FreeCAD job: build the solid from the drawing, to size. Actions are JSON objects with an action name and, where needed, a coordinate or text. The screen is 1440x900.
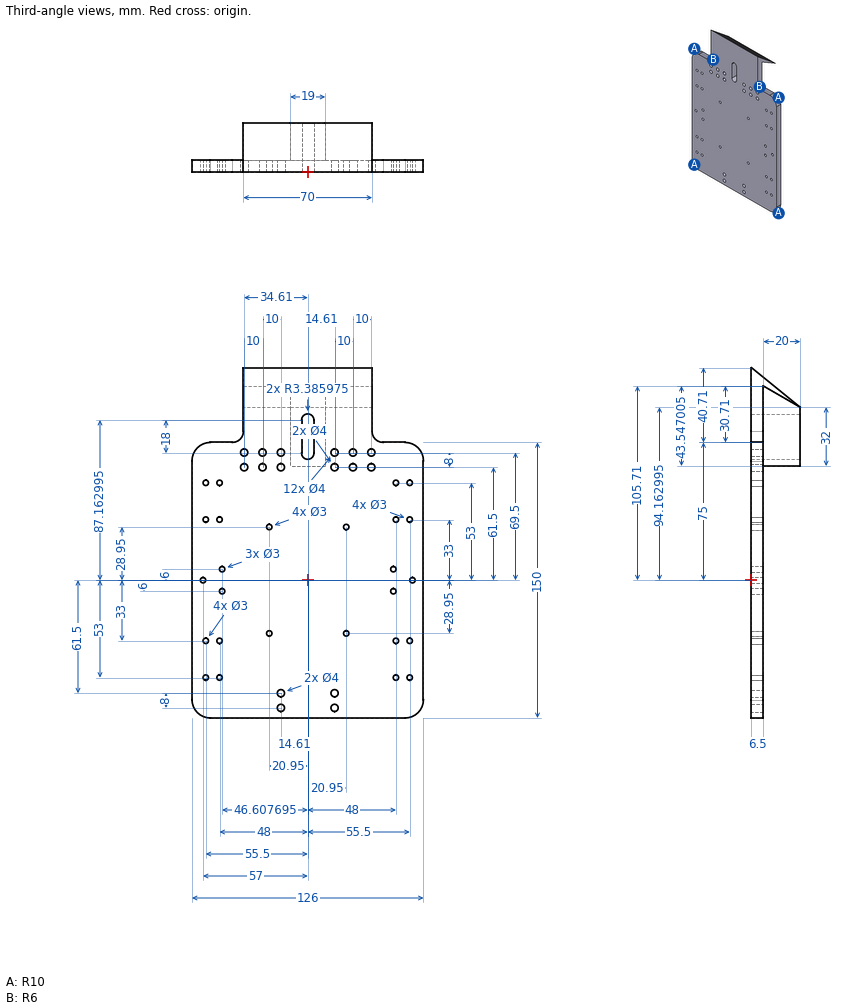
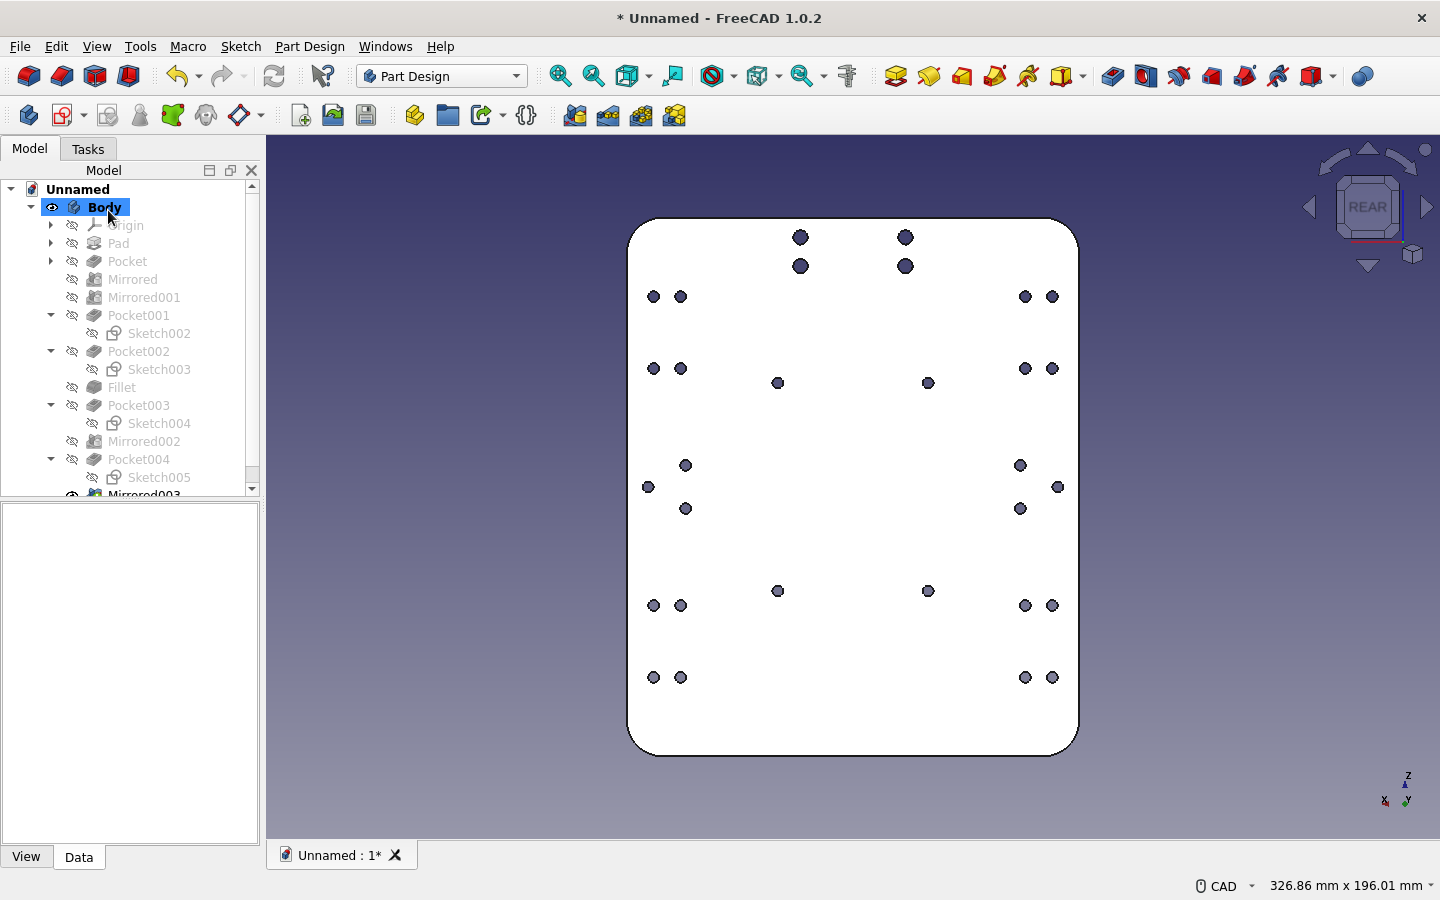
{"action": "left_click", "coordinate": [117, 459]}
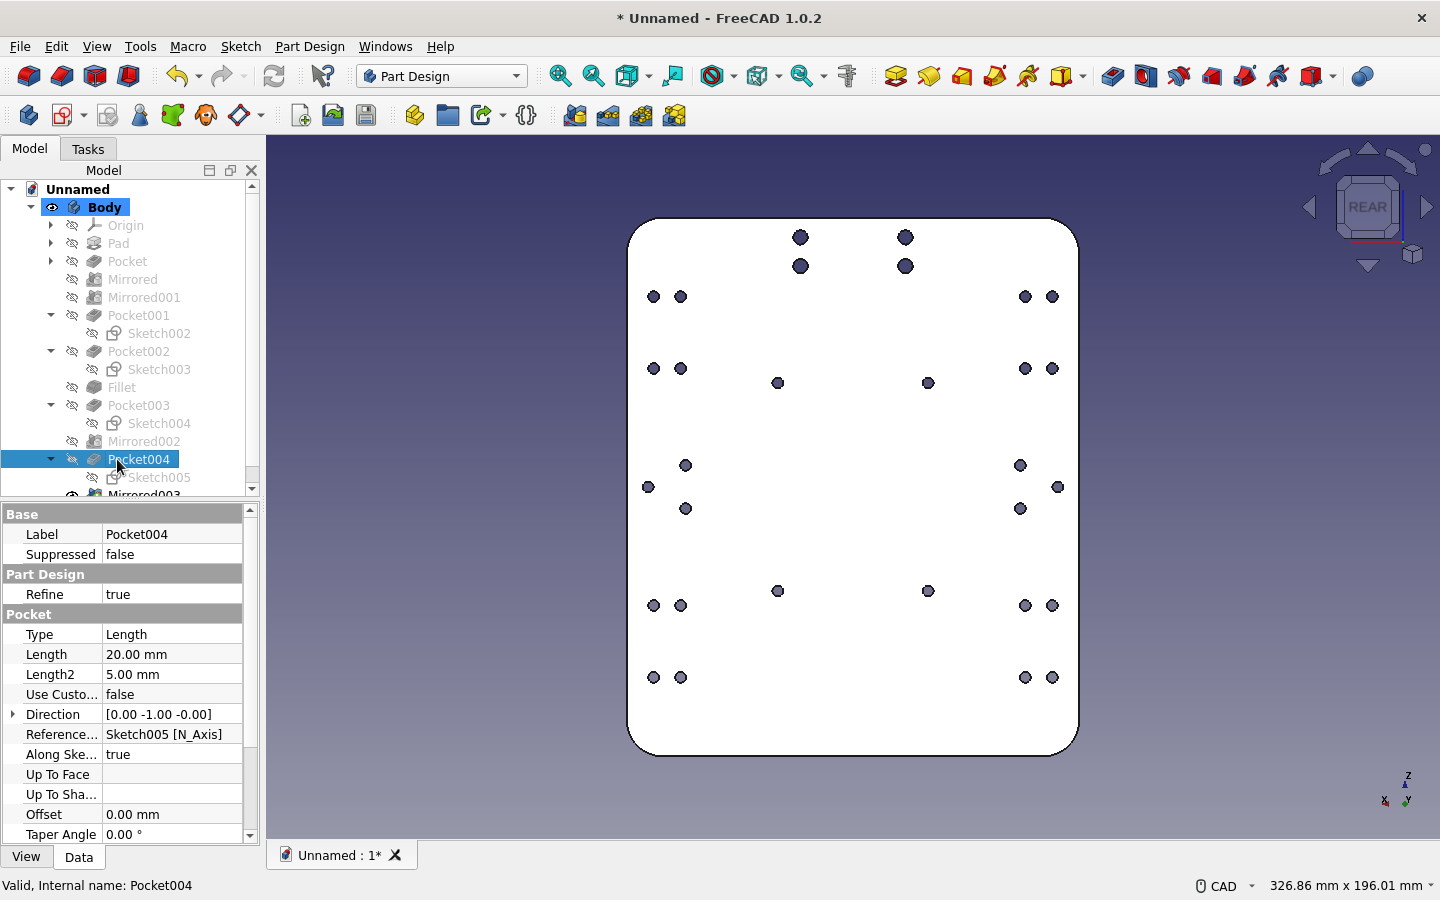
{"action": "left_click", "coordinate": [575, 116]}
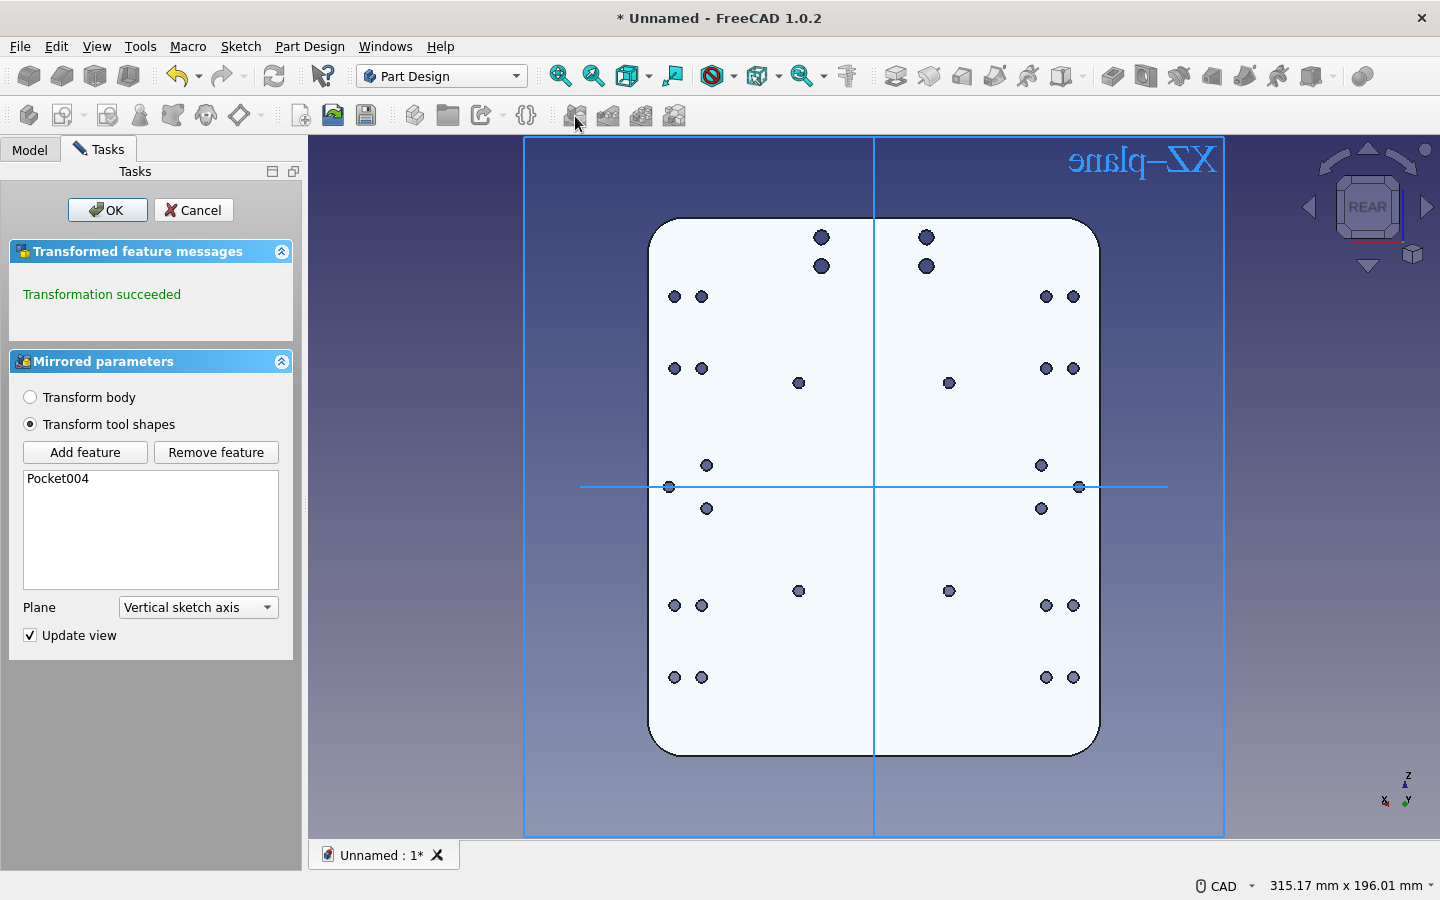
{"action": "left_click", "coordinate": [199, 608]}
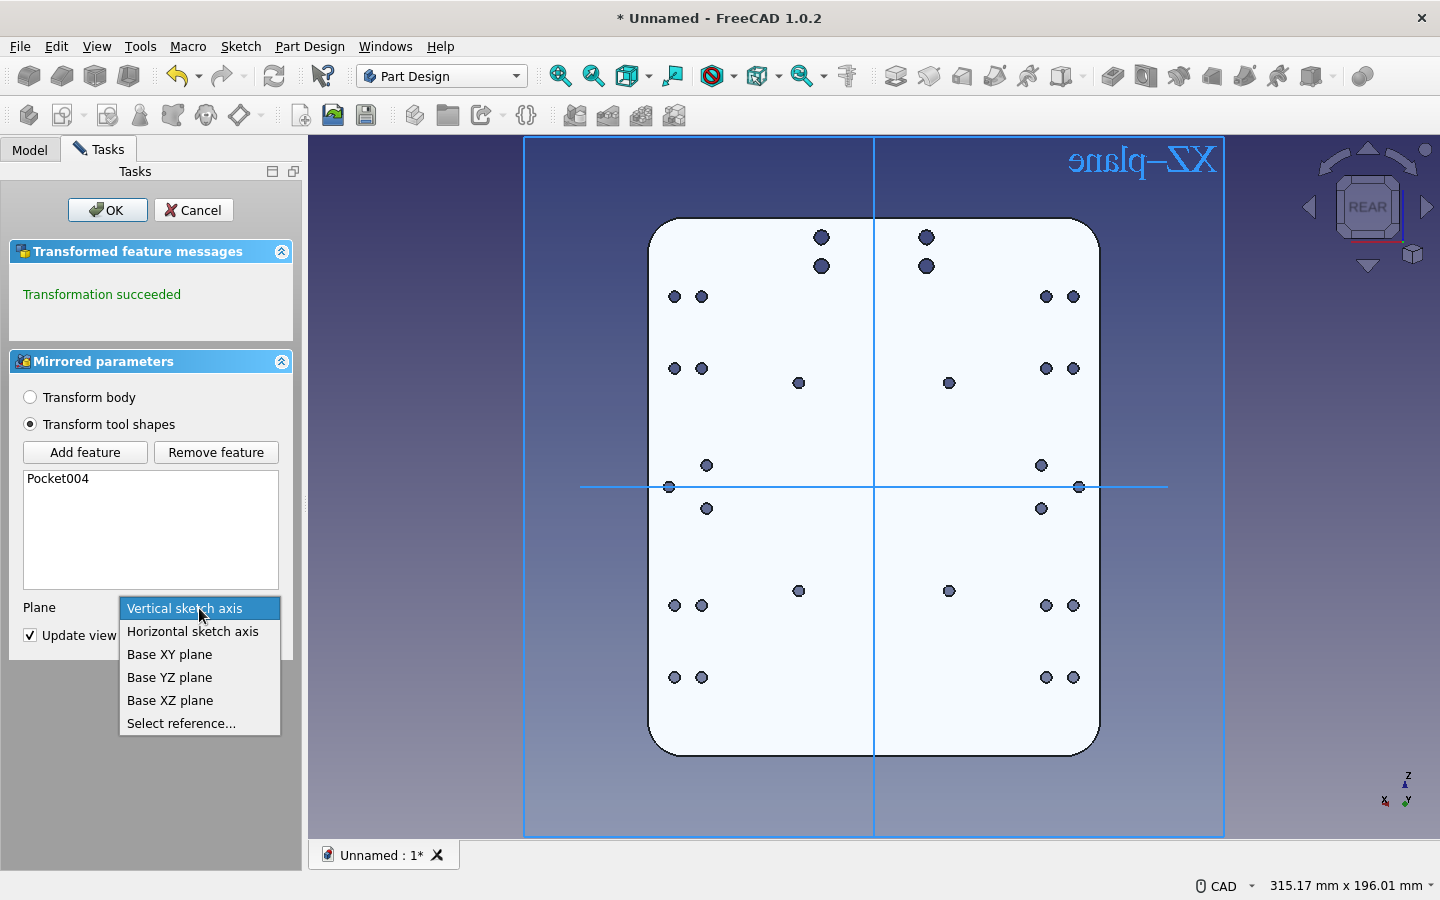
{"action": "left_click", "coordinate": [198, 654]}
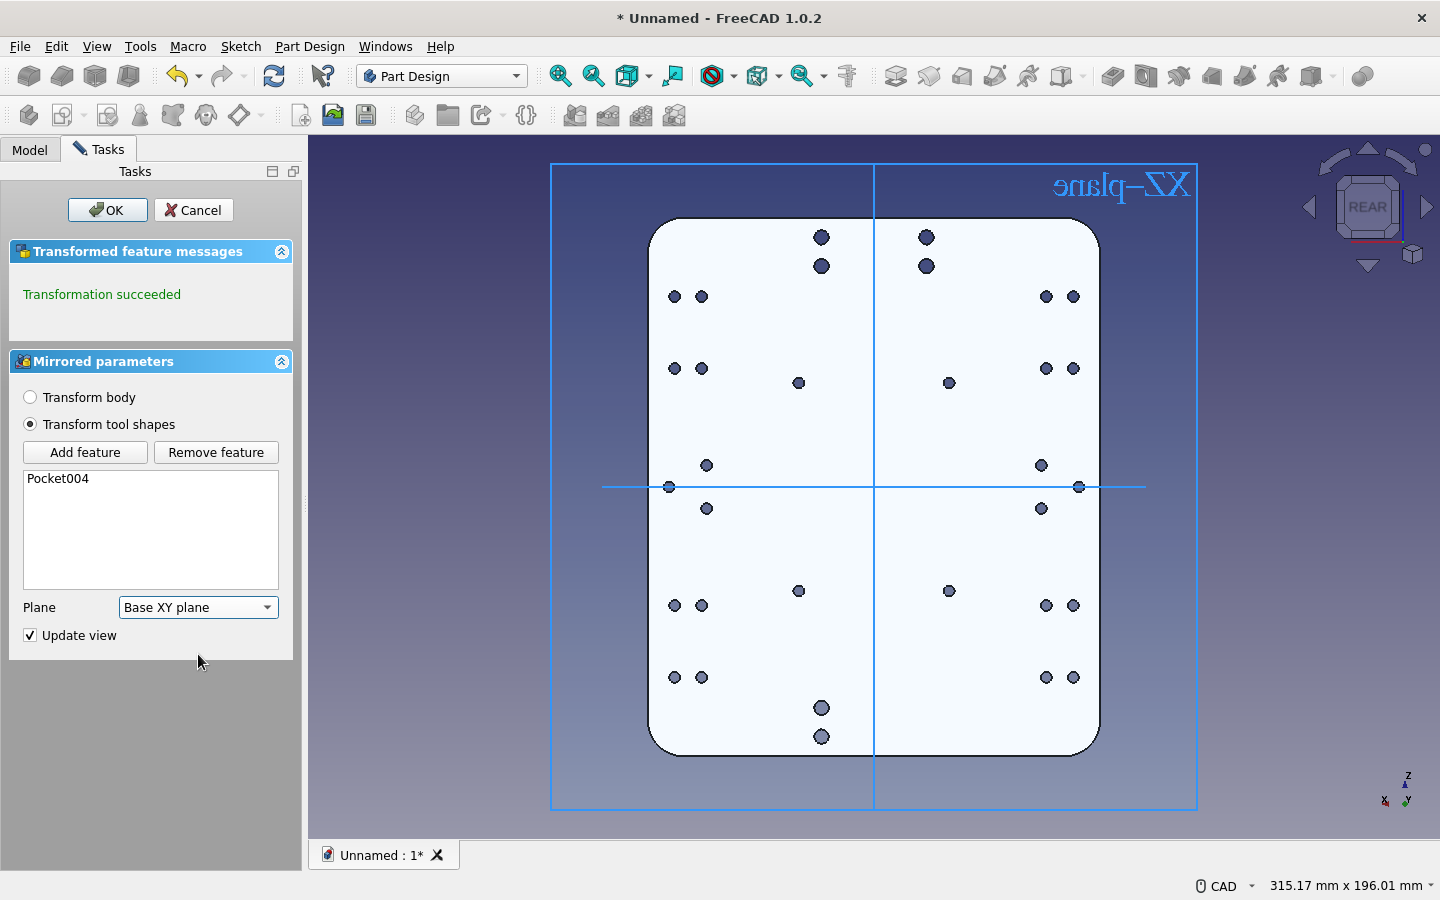
{"action": "left_click", "coordinate": [108, 210]}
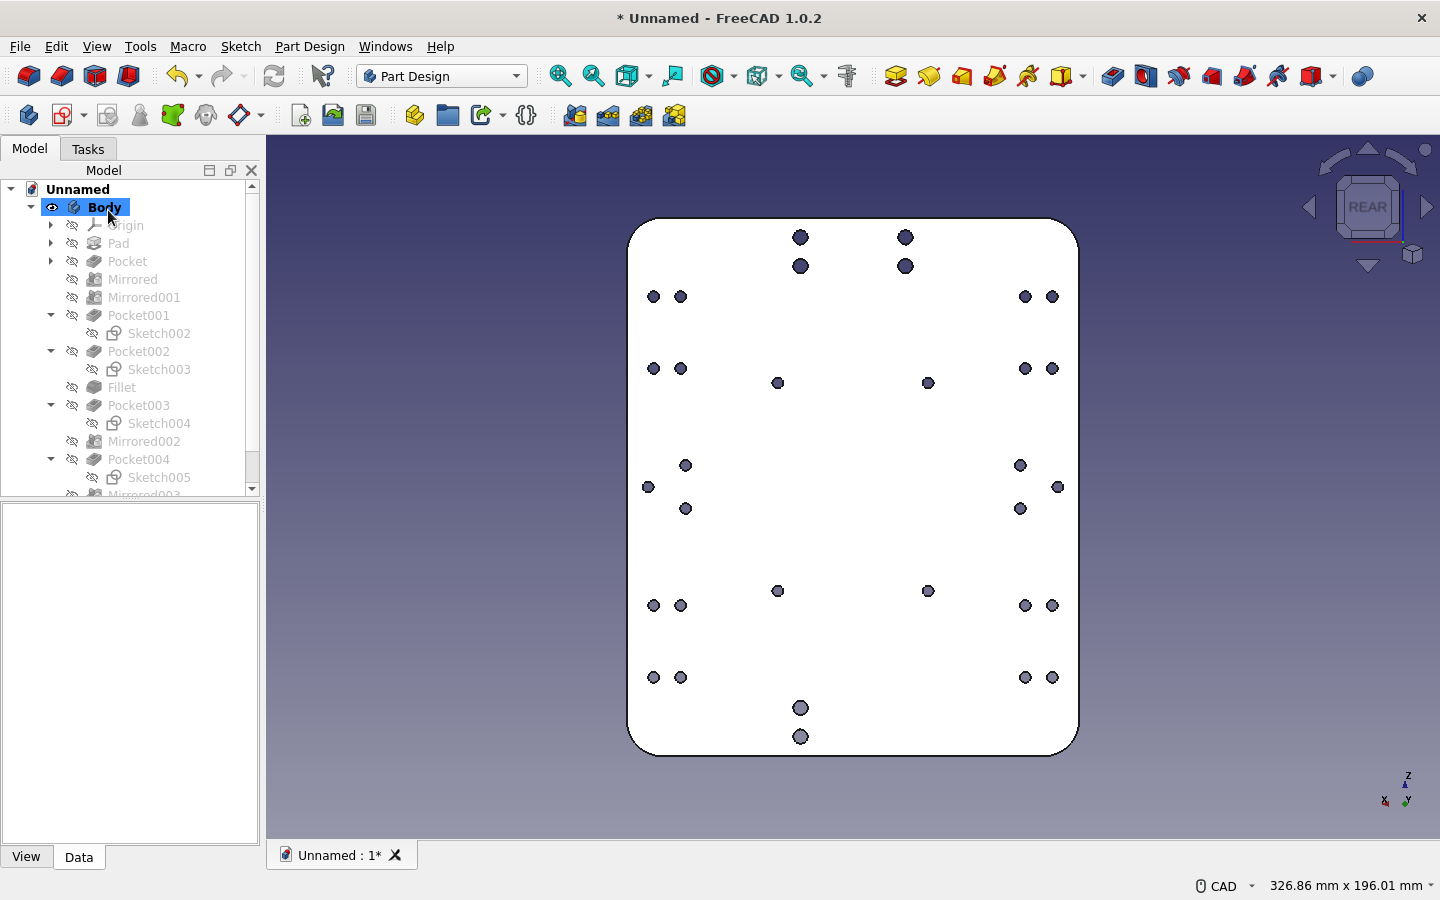
{"action": "left_click", "coordinate": [853, 486]}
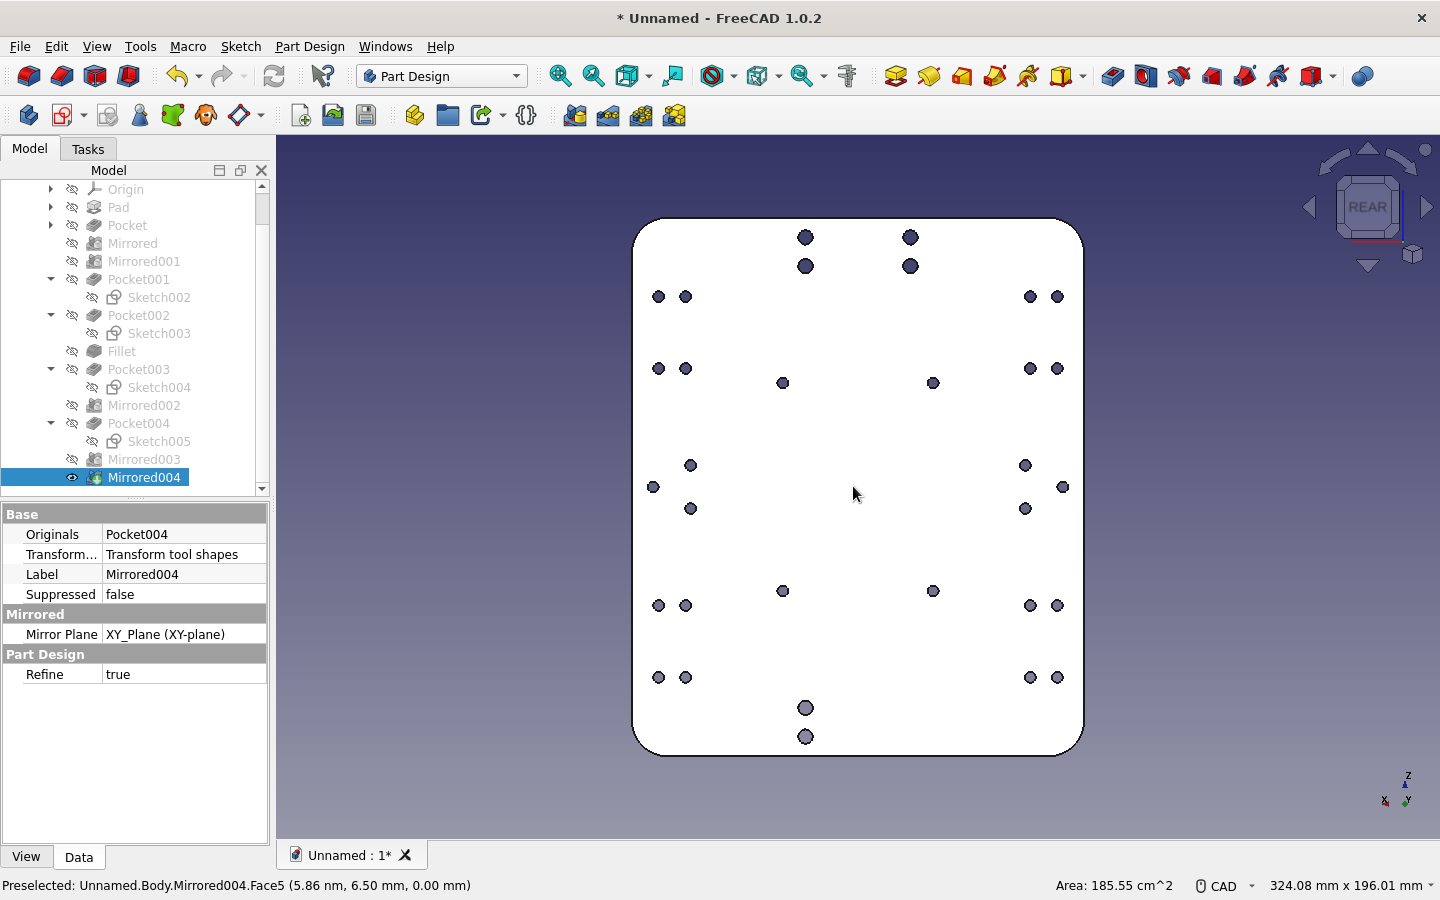
{"action": "left_click", "coordinate": [62, 116]}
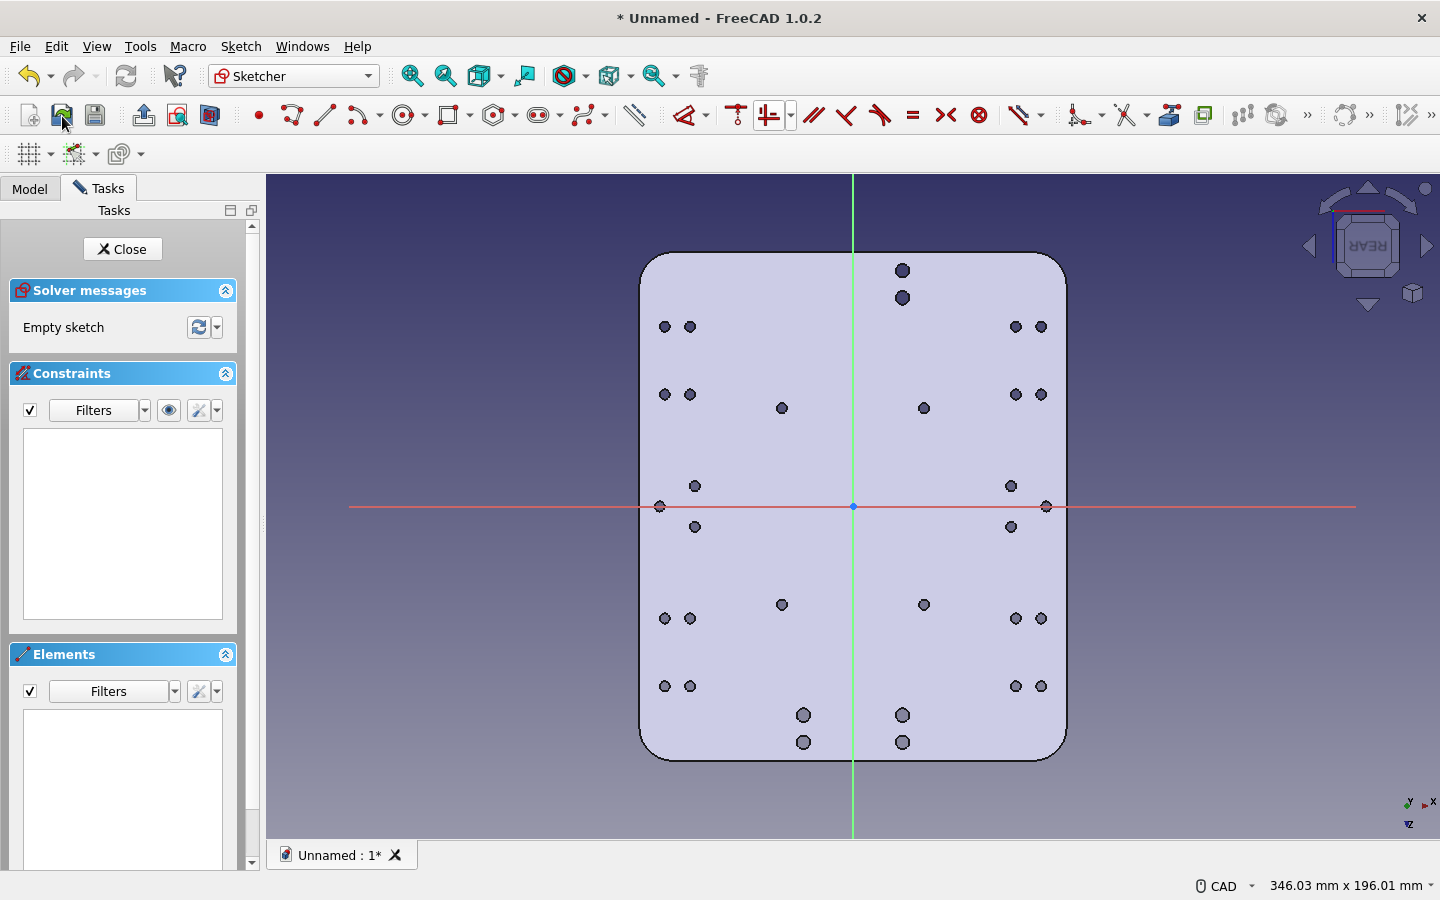
{"action": "scroll", "coordinate": [805, 262], "scroll_direction": "up", "scroll_amount": 12}